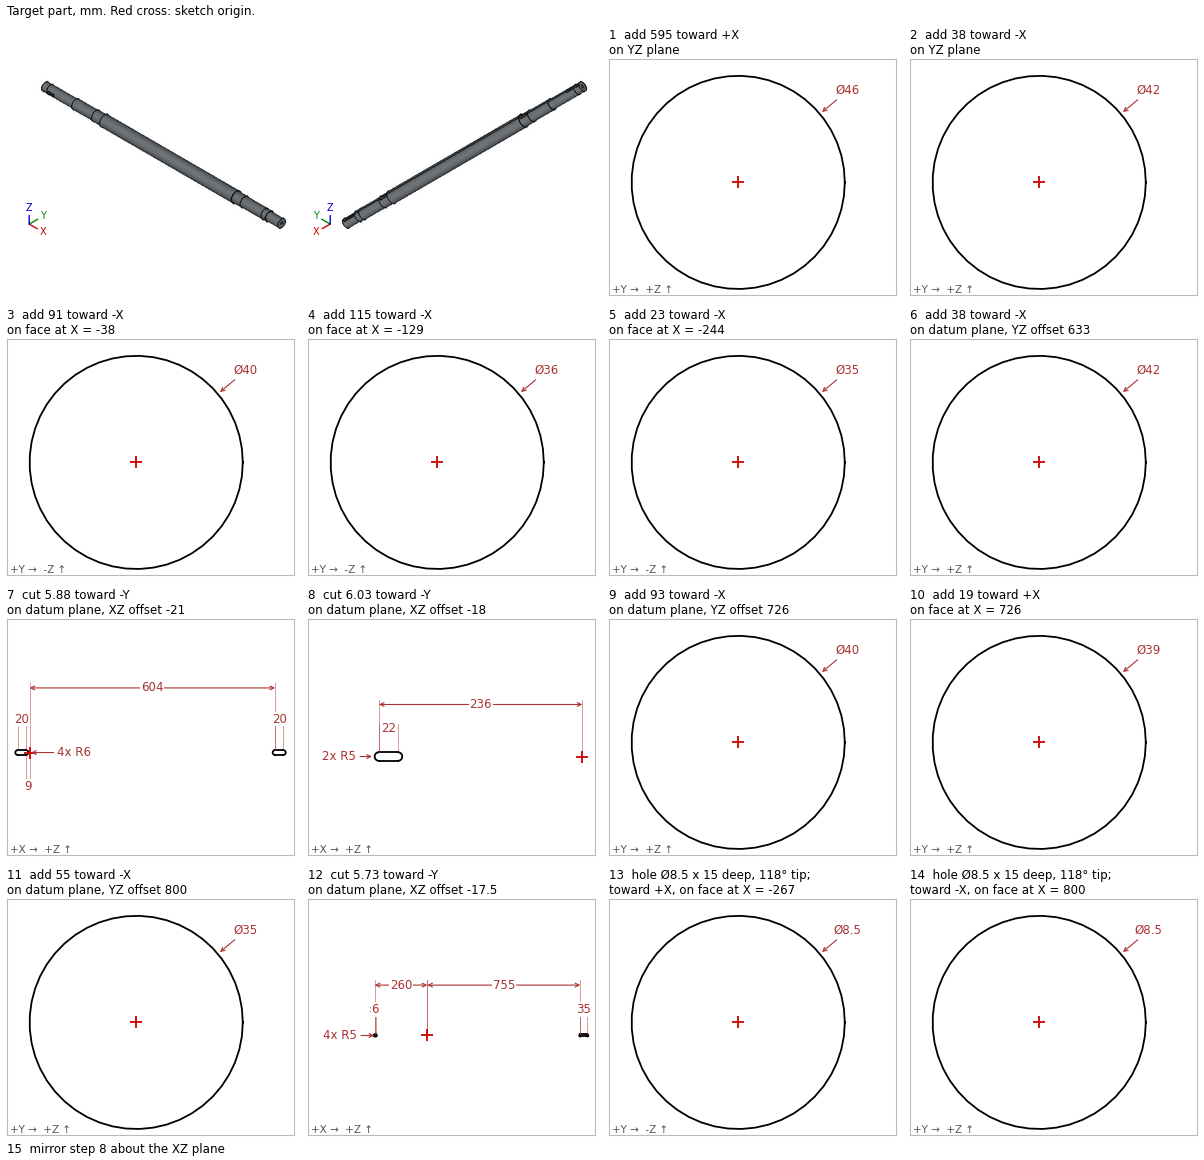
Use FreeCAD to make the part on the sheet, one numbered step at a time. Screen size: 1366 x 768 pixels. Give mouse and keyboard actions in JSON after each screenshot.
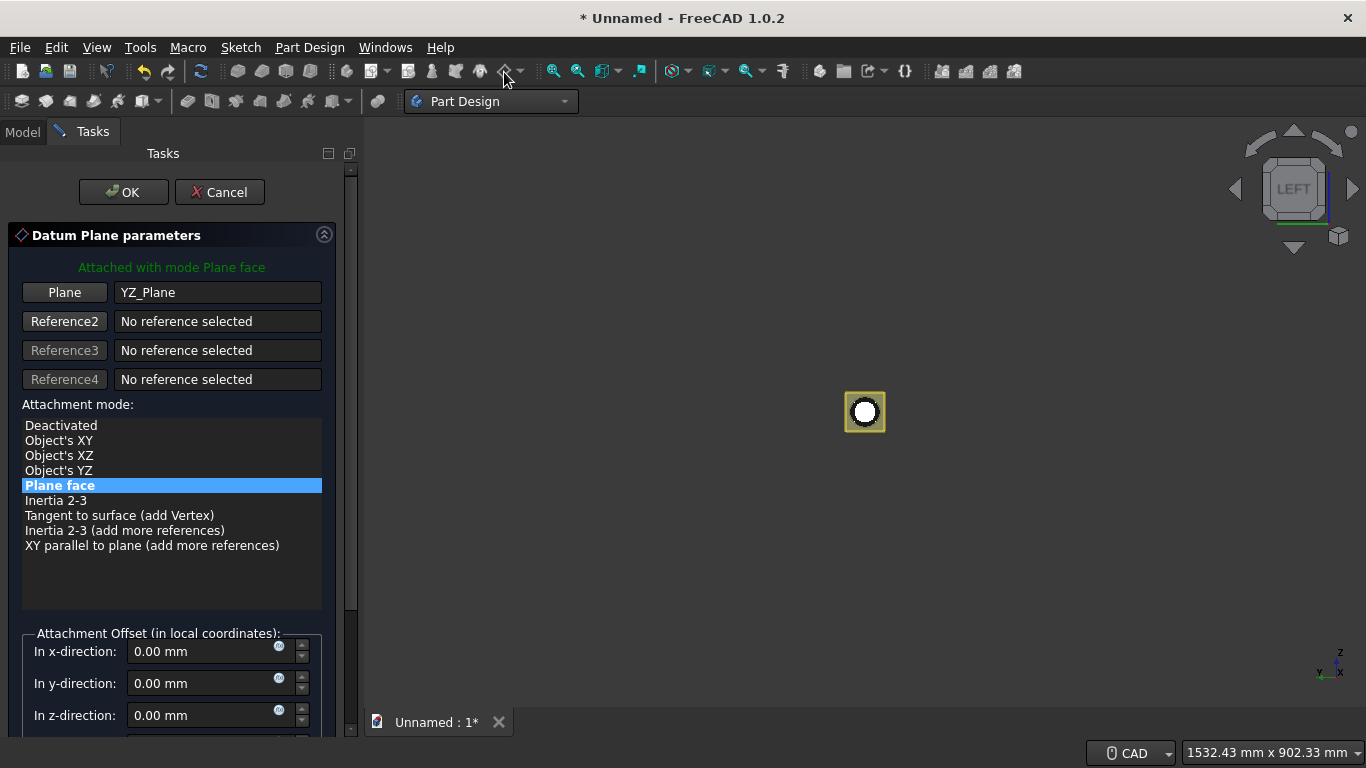
{"action": "triple_click", "coordinate": [210, 715]}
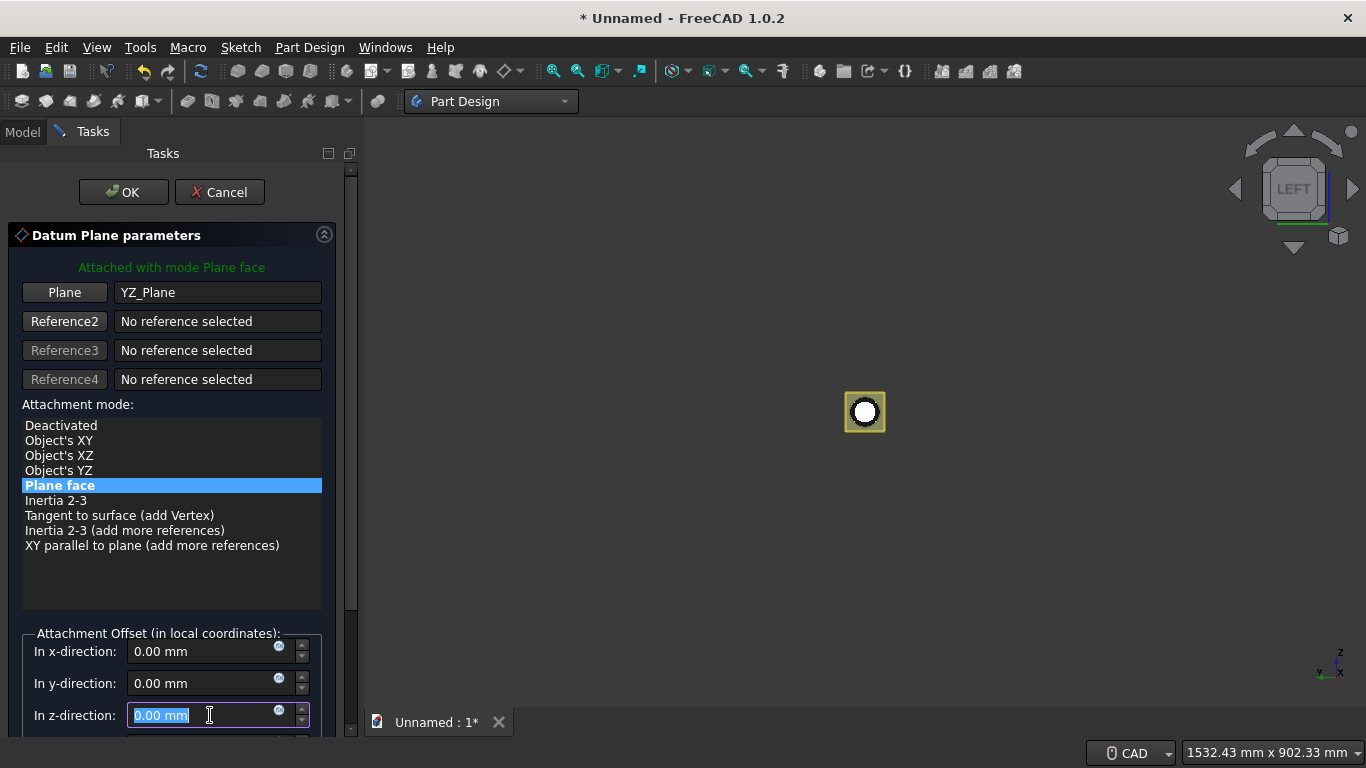
{"action": "type", "text": "726"}
{"action": "key", "text": "Tab"}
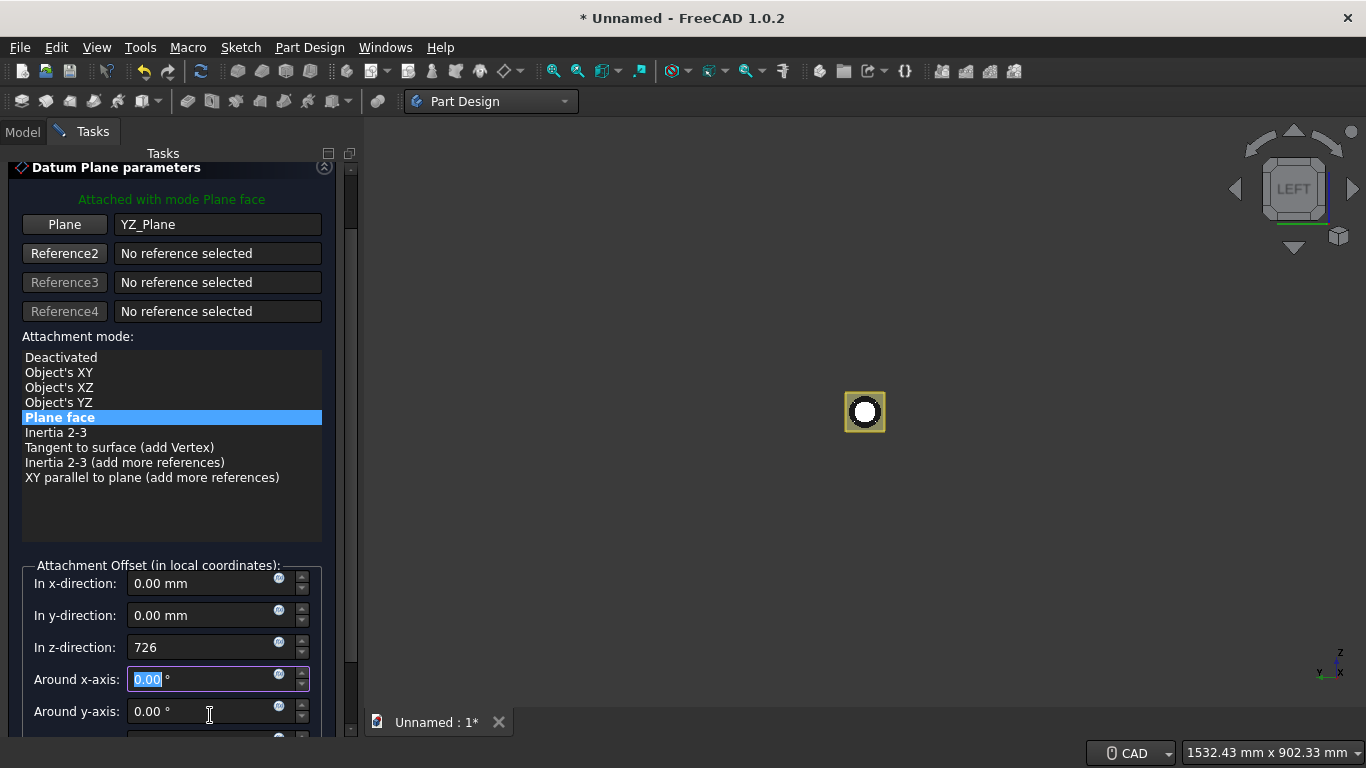
{"action": "scroll", "coordinate": [351, 450], "scroll_direction": "up", "scroll_amount": 2}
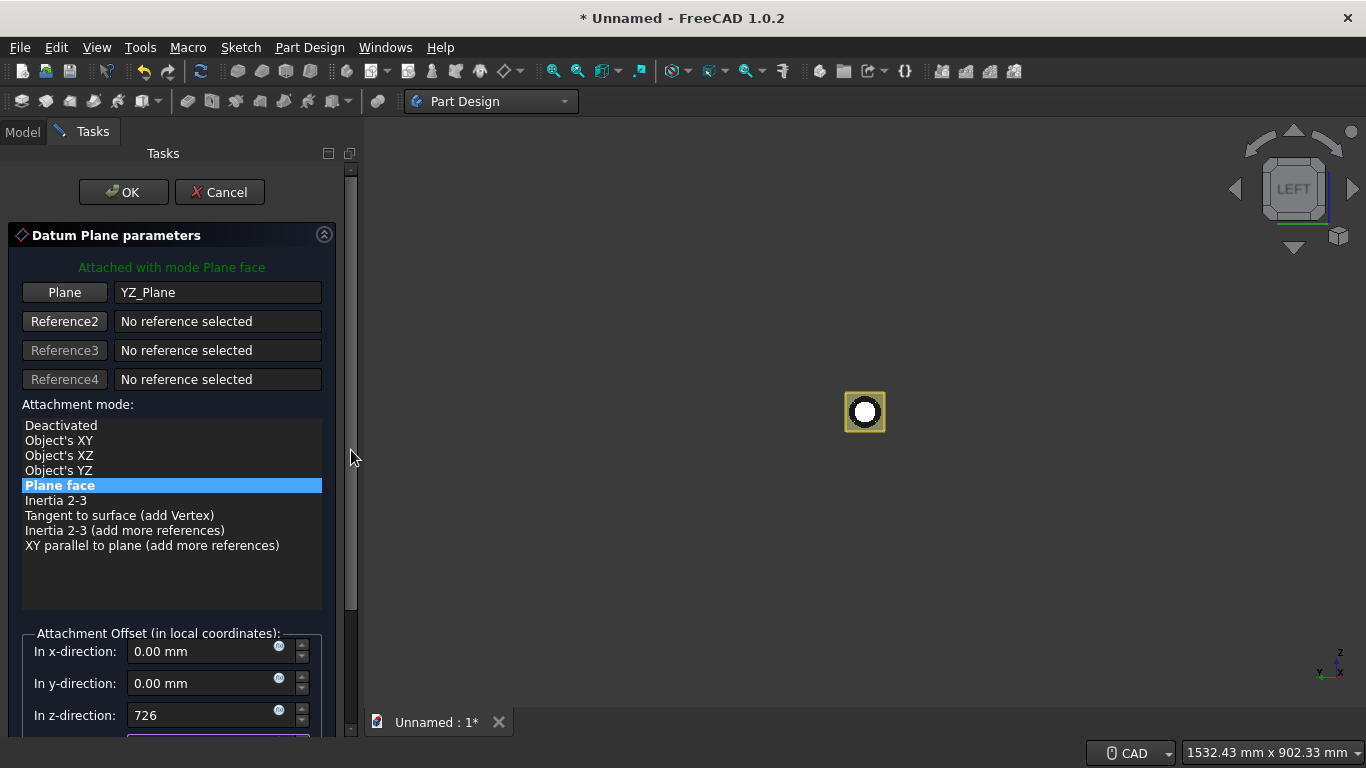
{"action": "left_click", "coordinate": [124, 192]}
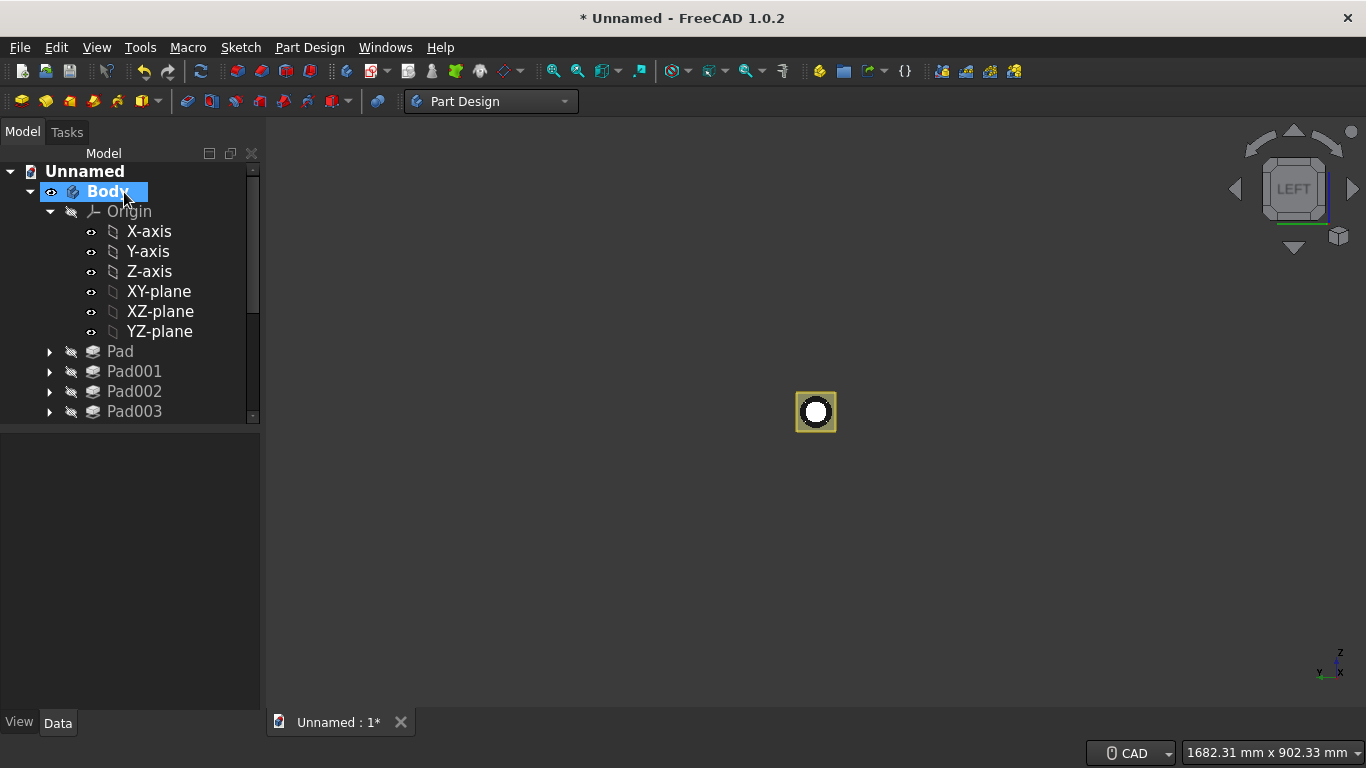
{"action": "scroll", "coordinate": [100, 287], "scroll_direction": "down", "scroll_amount": 3}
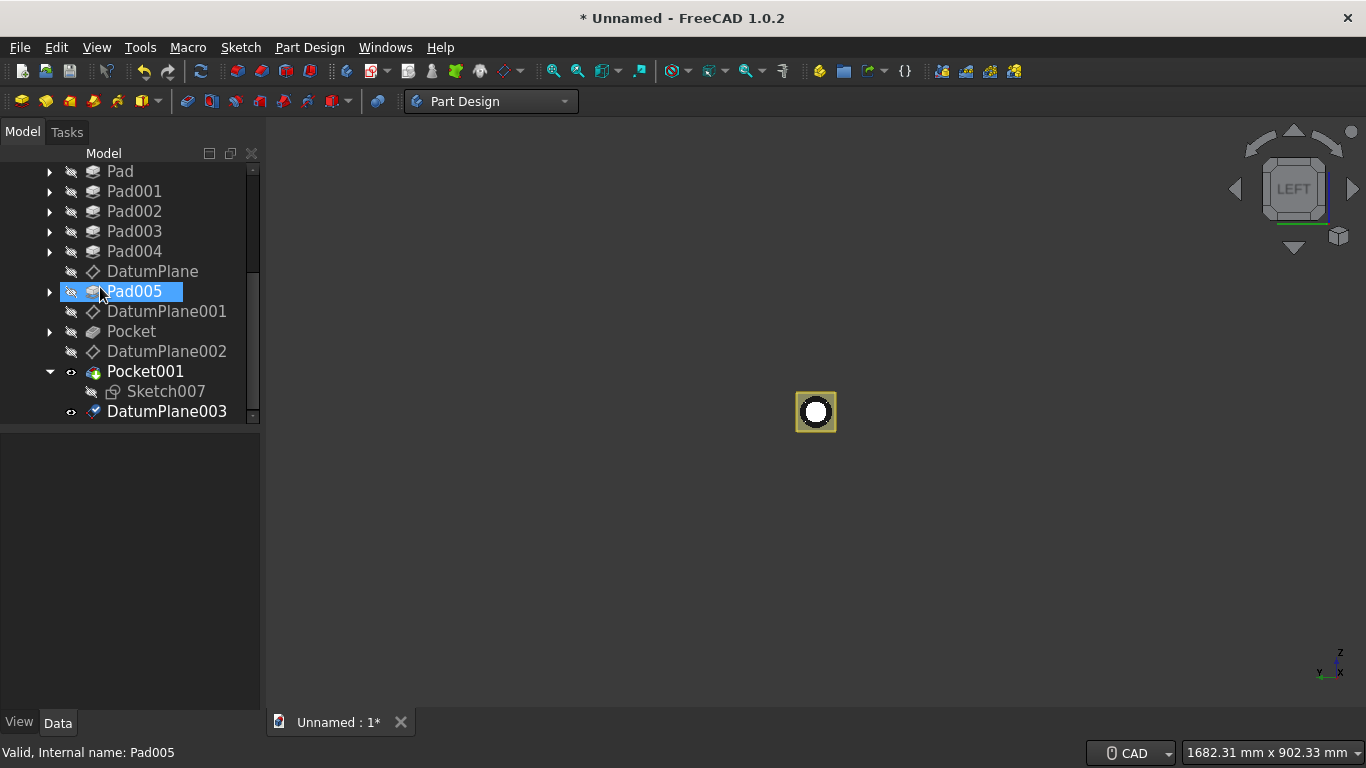
{"action": "left_click", "coordinate": [116, 412]}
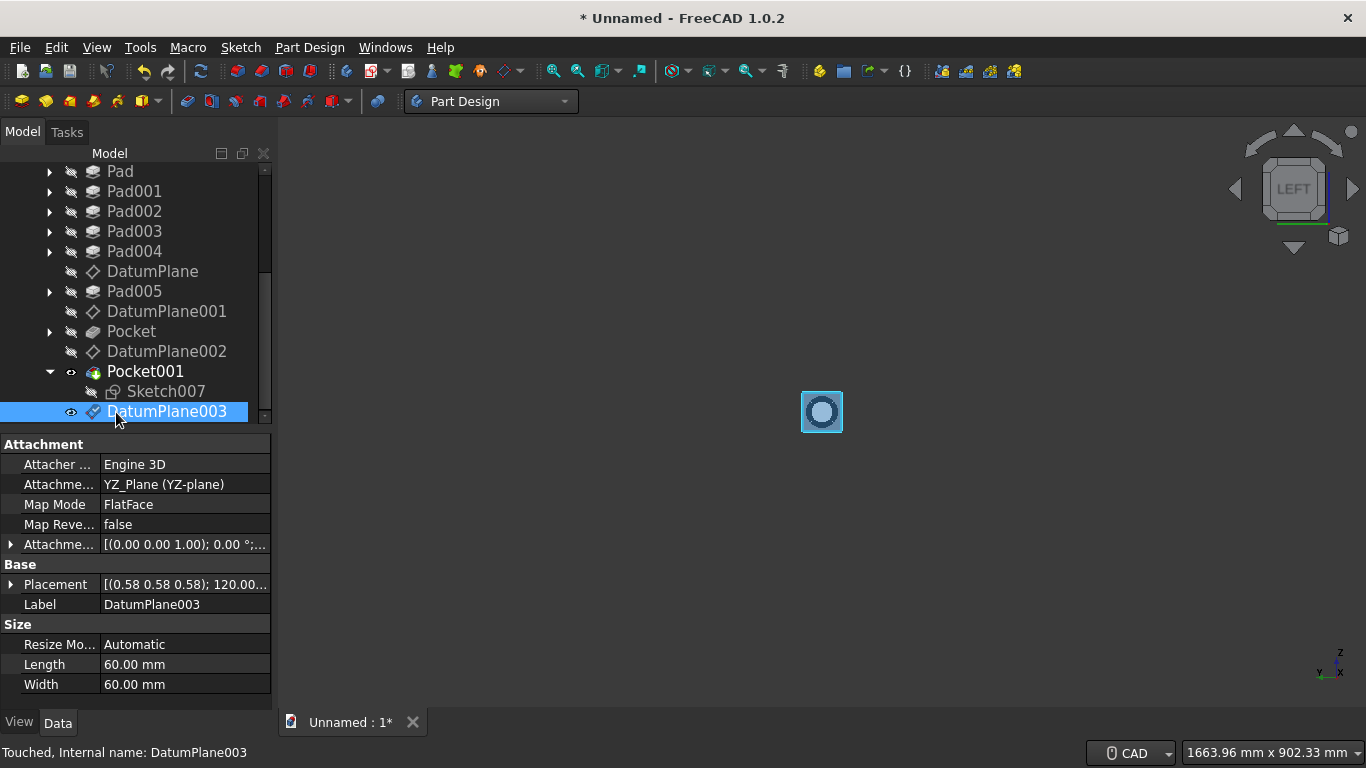
{"action": "left_click", "coordinate": [372, 72]}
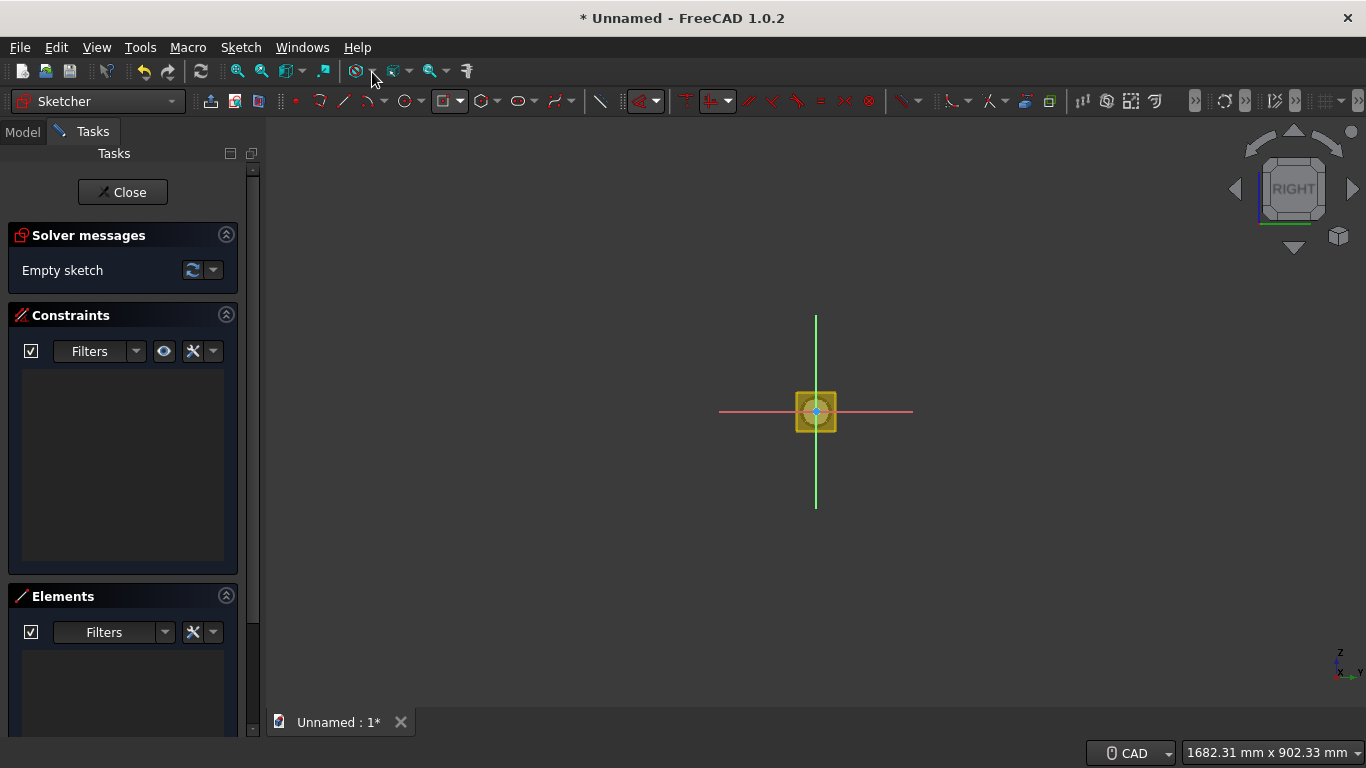
{"action": "scroll", "coordinate": [821, 412], "scroll_direction": "up", "scroll_amount": 13}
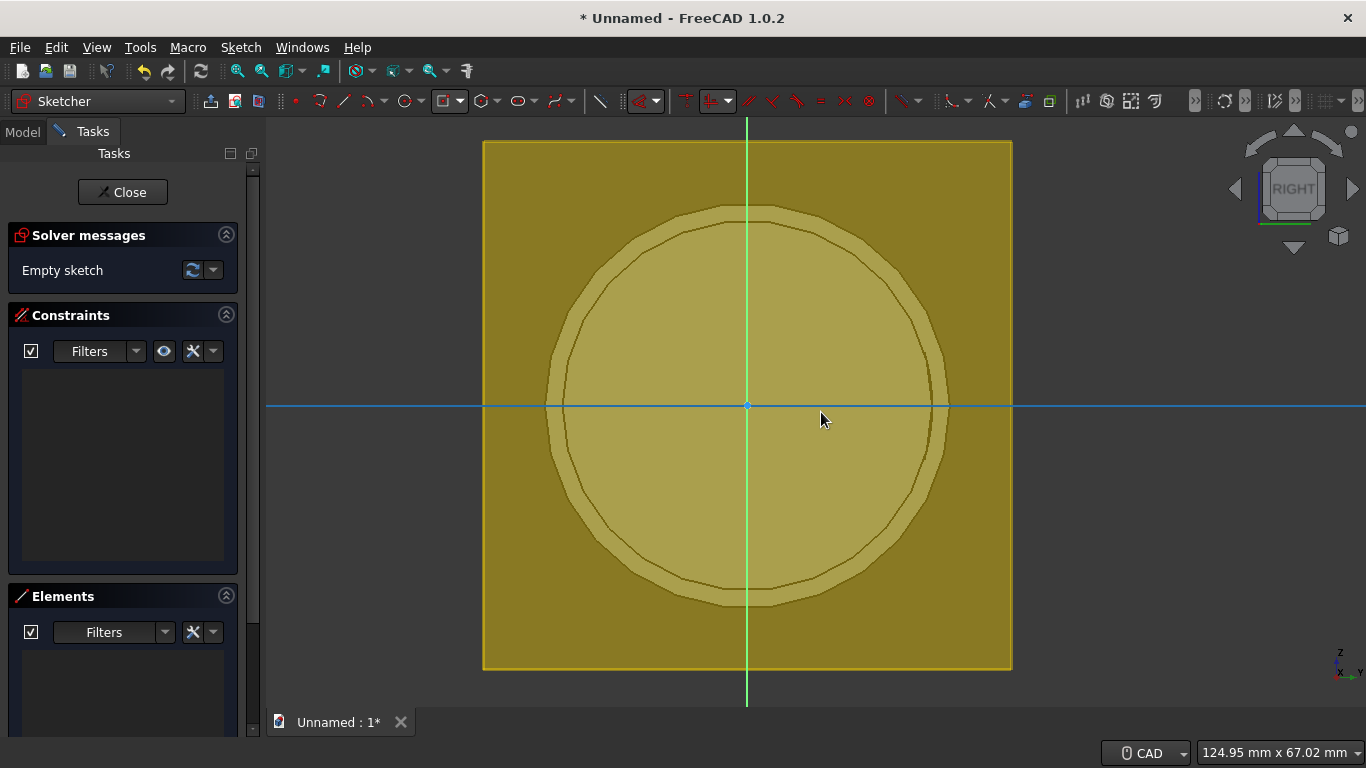
{"action": "key", "text": "g c"}